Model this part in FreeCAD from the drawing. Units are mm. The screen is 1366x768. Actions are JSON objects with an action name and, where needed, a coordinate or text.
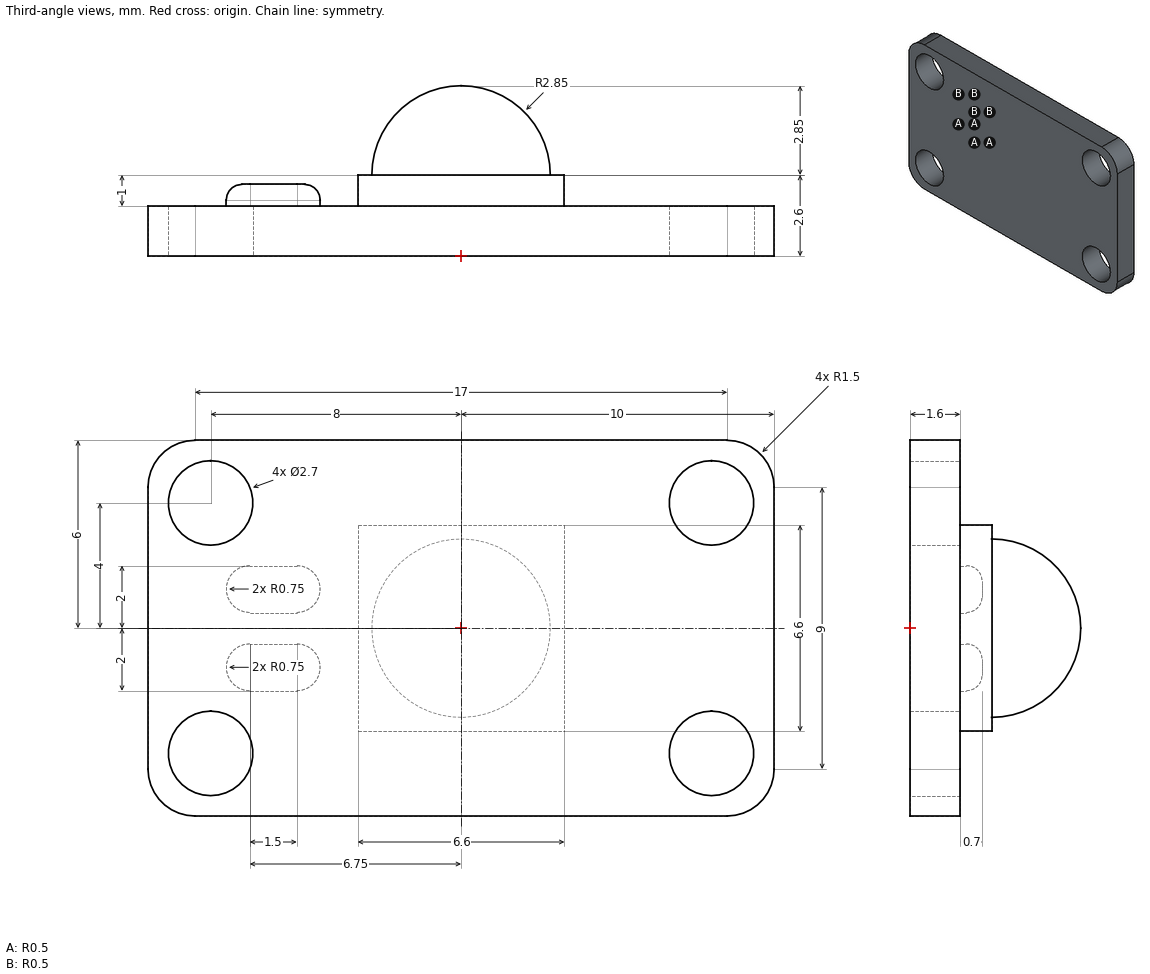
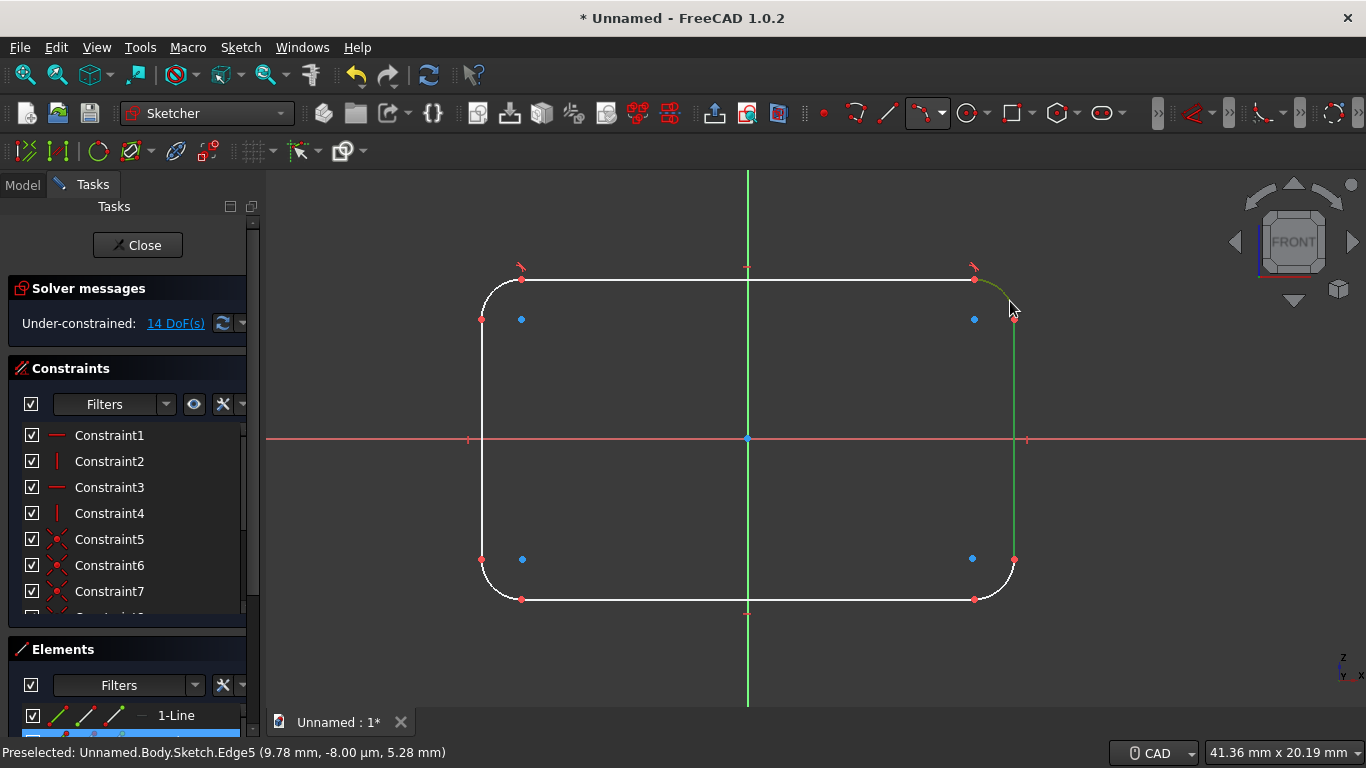
{"action": "key", "text": "t"}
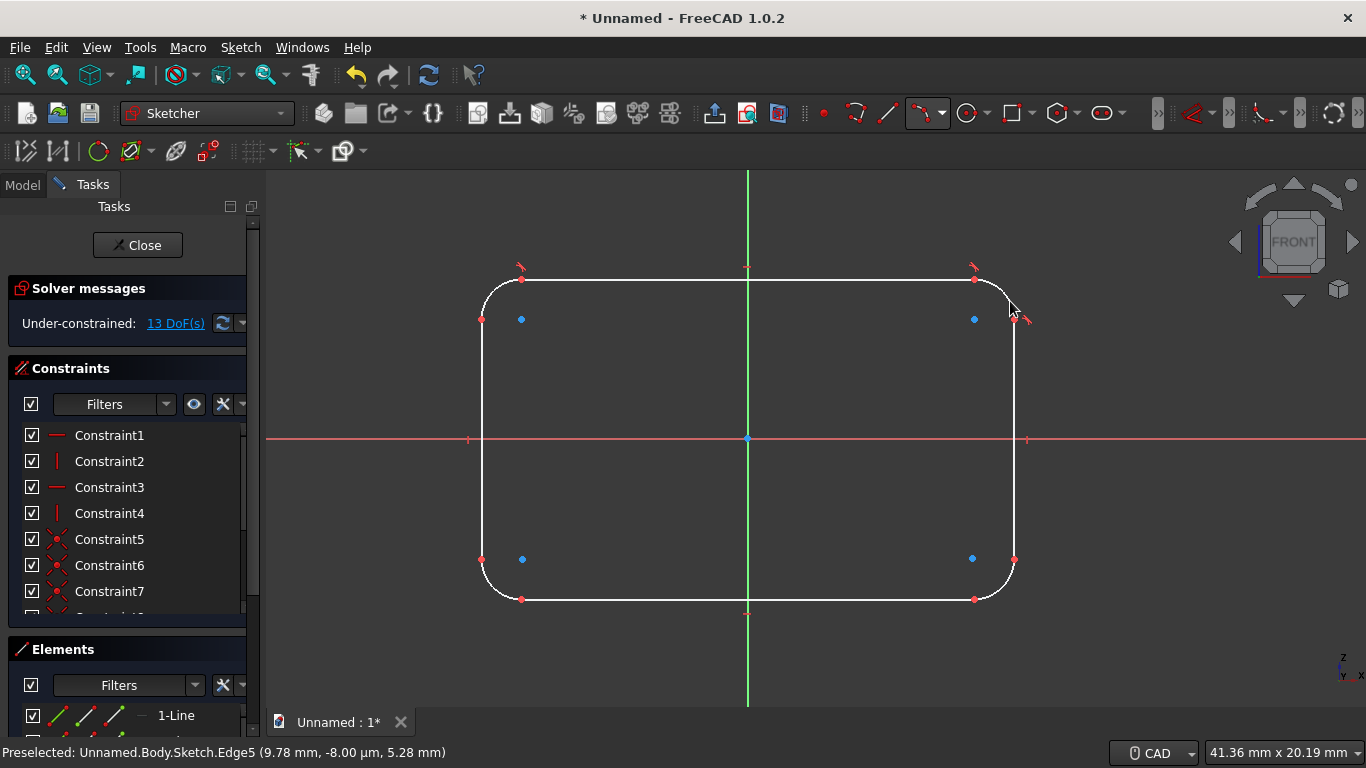
{"action": "left_click", "coordinate": [1014, 392]}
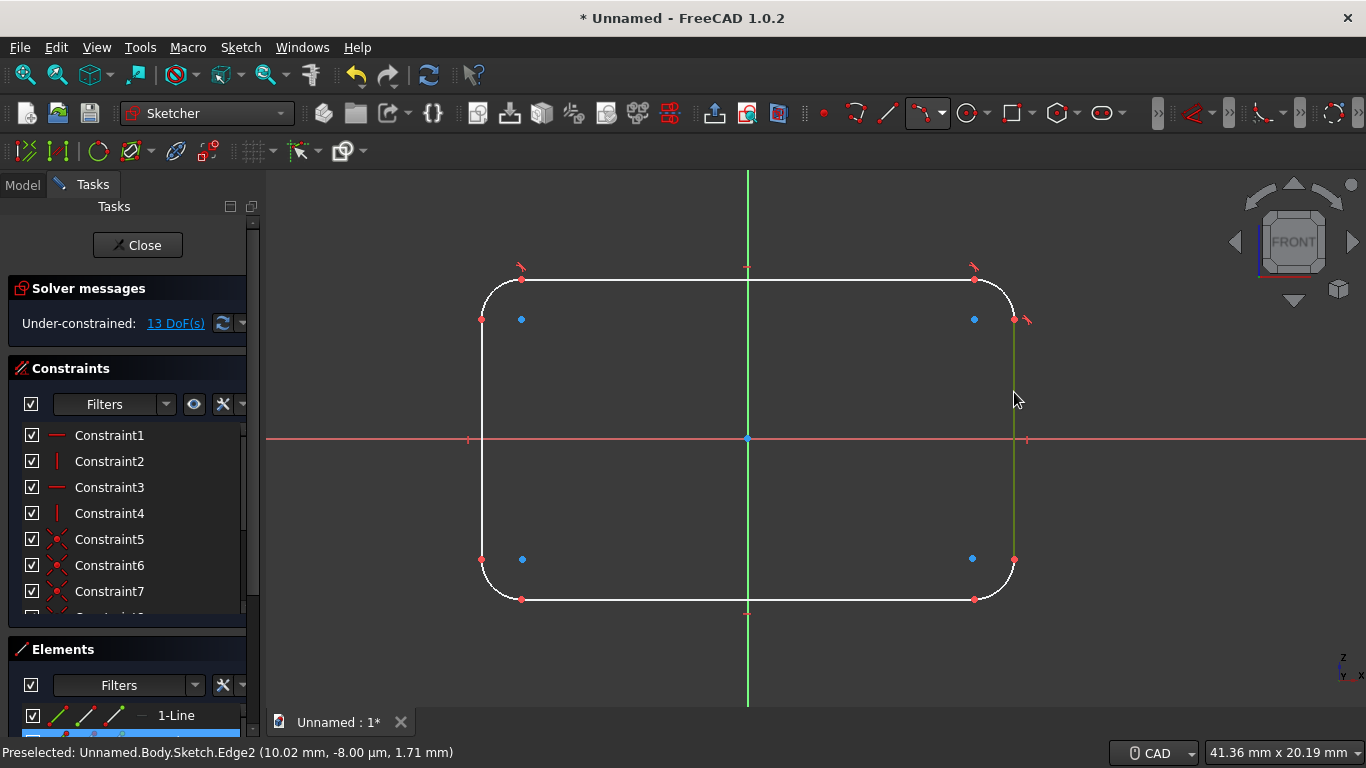
{"action": "left_click", "coordinate": [992, 595]}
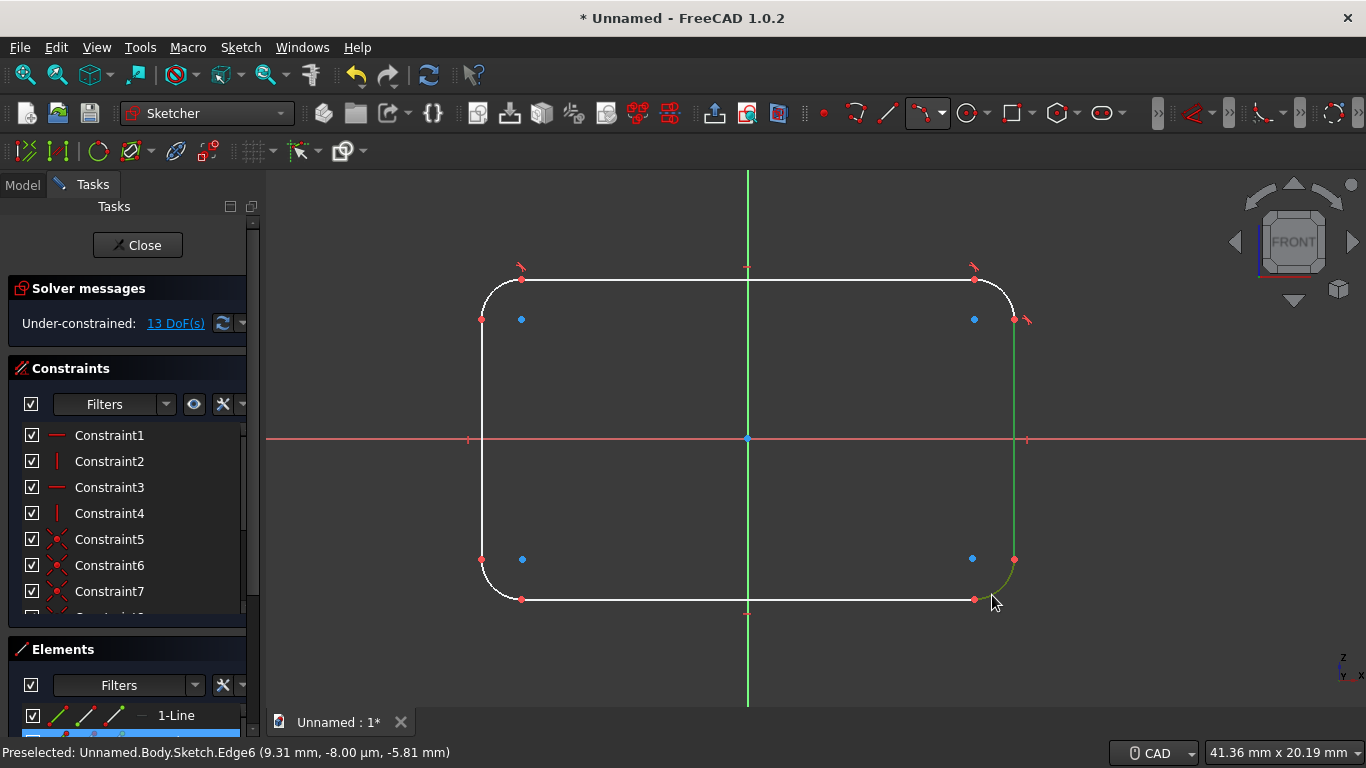
{"action": "key", "text": "t"}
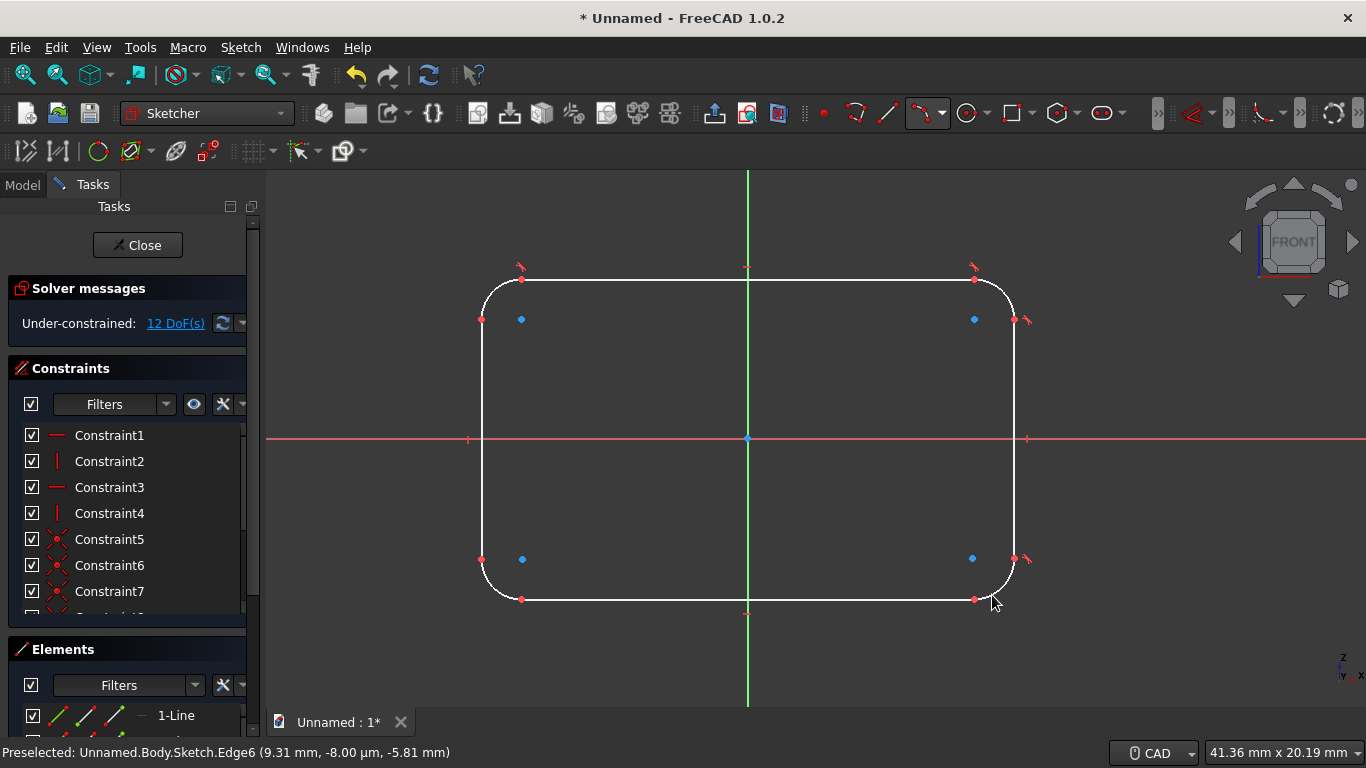
{"action": "left_click", "coordinate": [838, 600]}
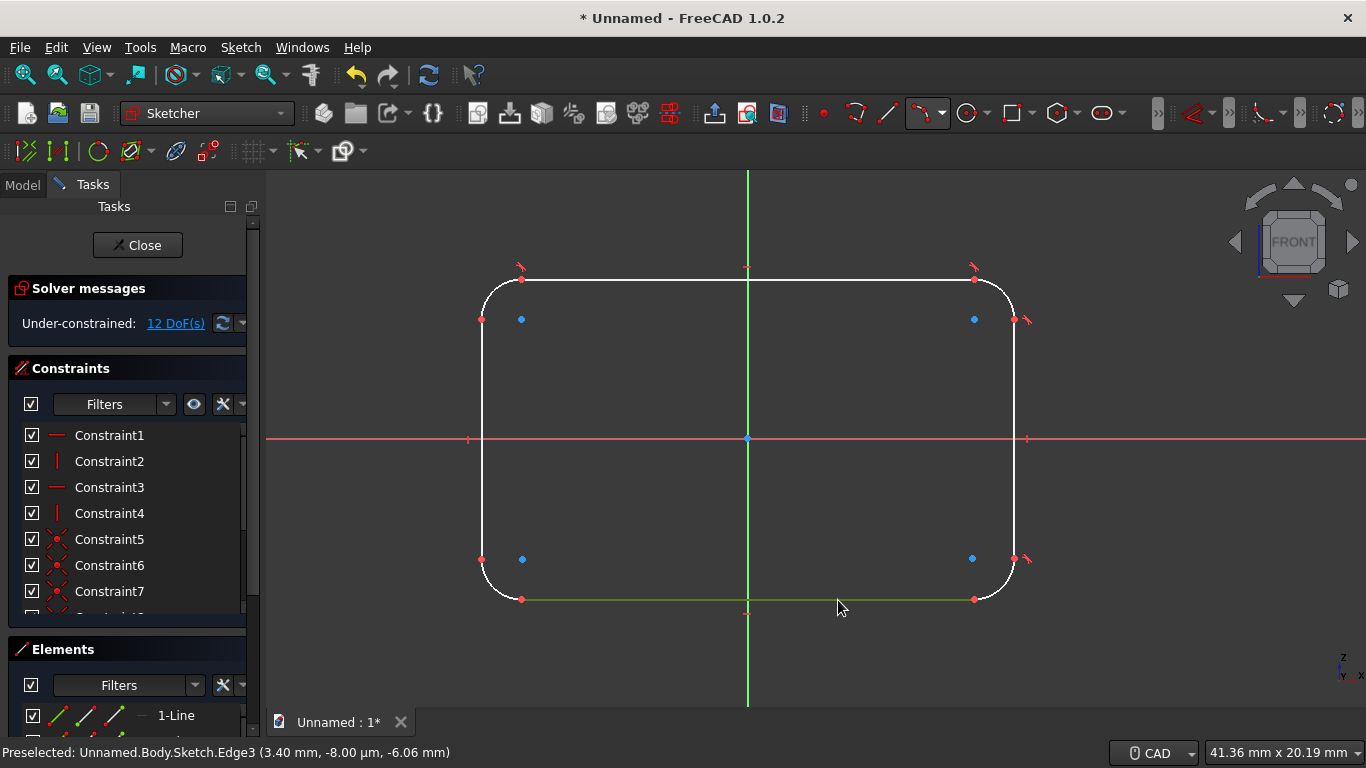
{"action": "left_click", "coordinate": [992, 595]}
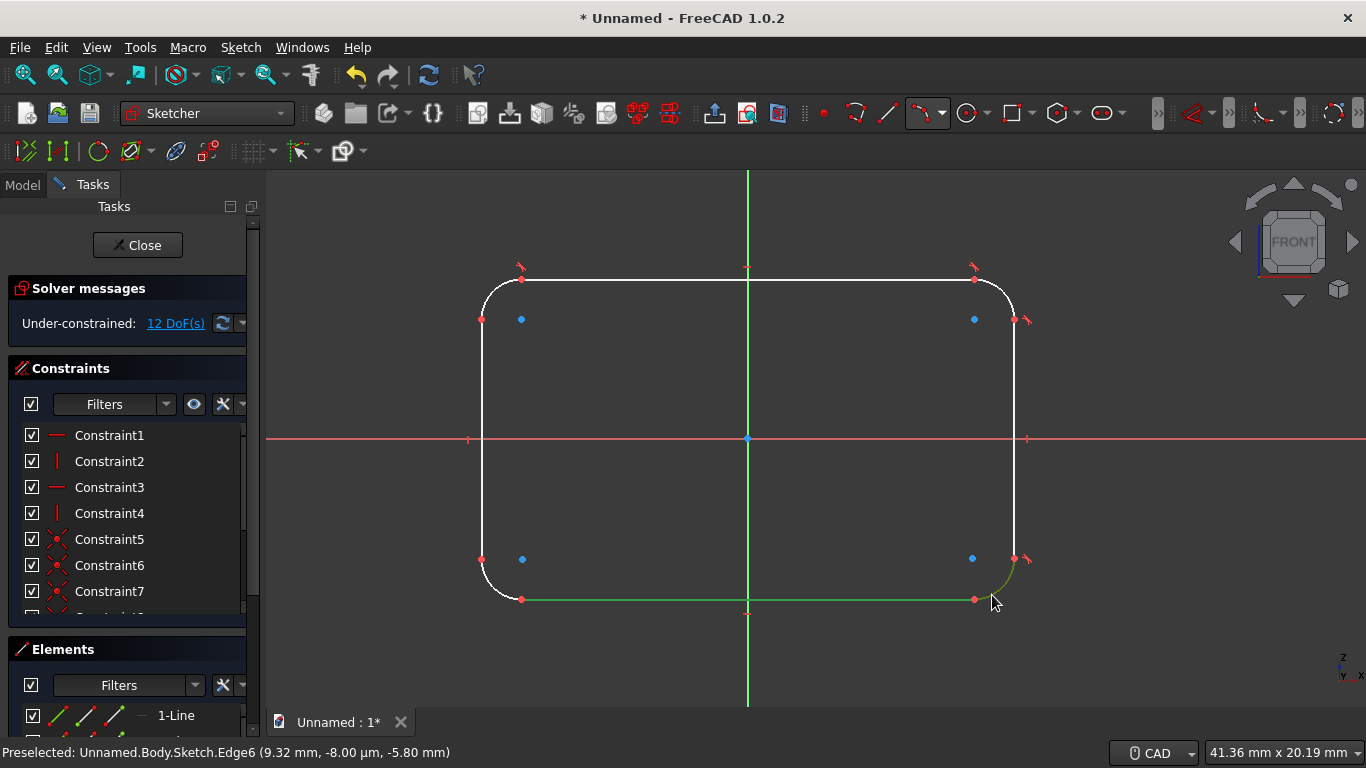
{"action": "key", "text": "t"}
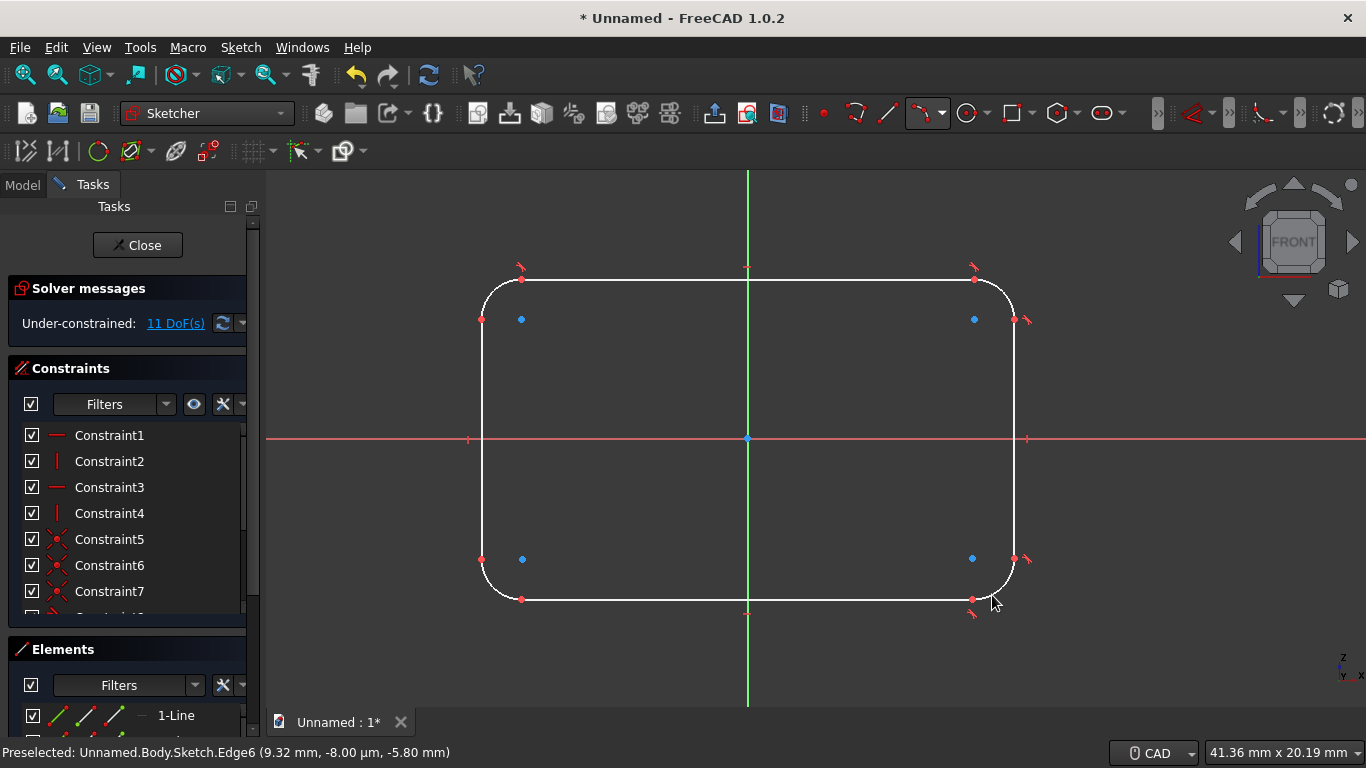
{"action": "left_click", "coordinate": [837, 600]}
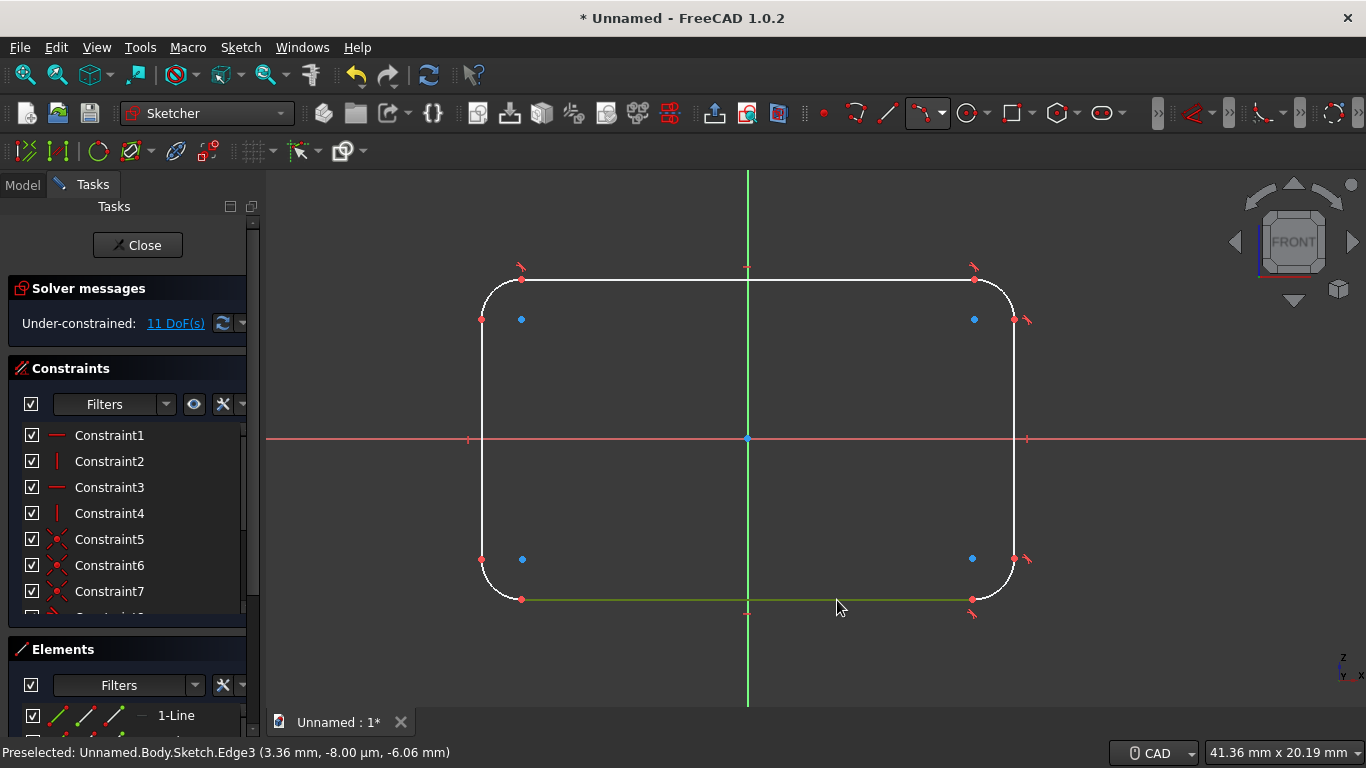
{"action": "left_click", "coordinate": [486, 578]}